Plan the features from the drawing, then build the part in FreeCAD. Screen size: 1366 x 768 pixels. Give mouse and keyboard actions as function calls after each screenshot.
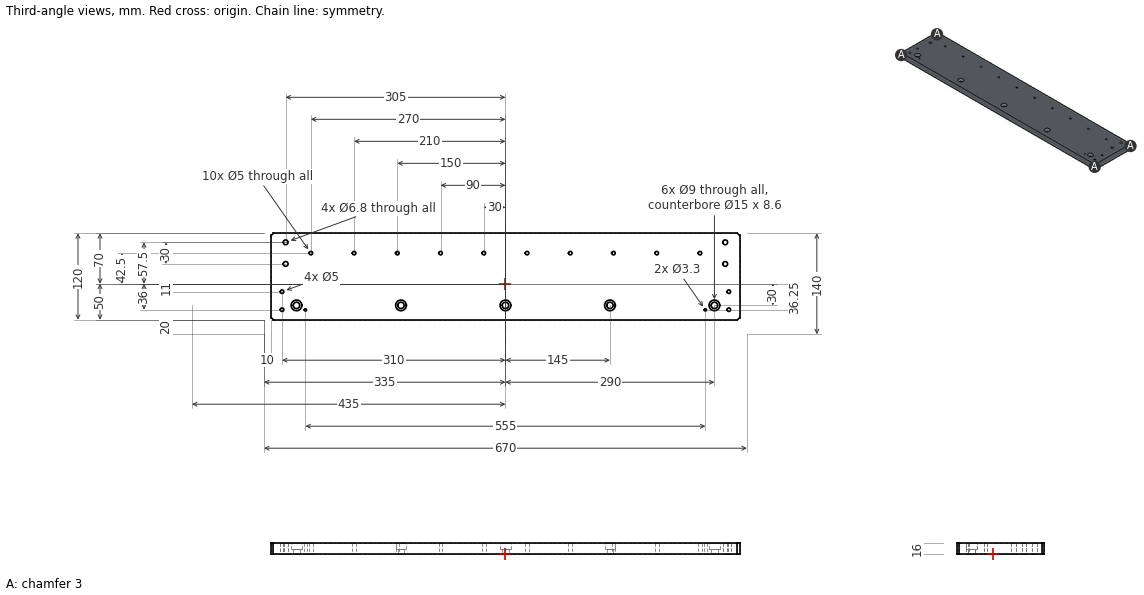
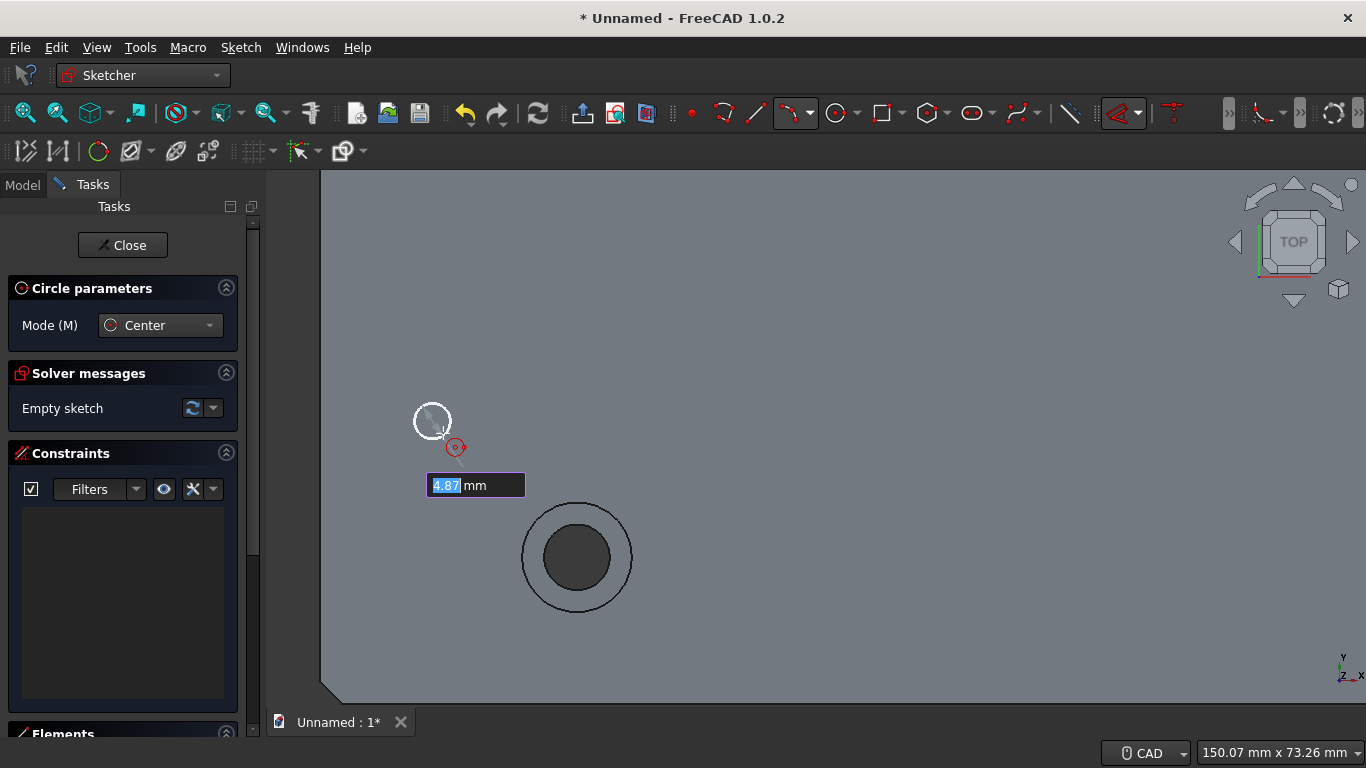
click(443, 431)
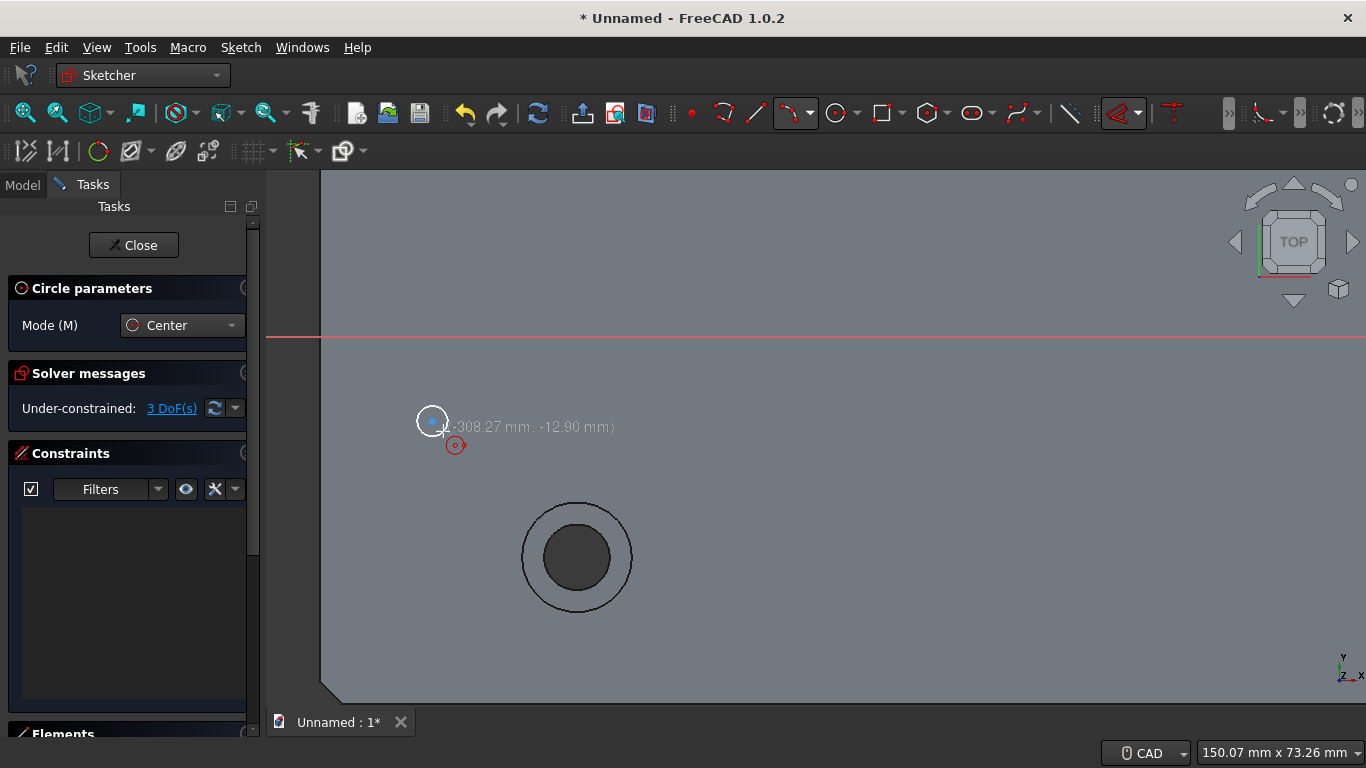
scroll(430, 601, up, 2)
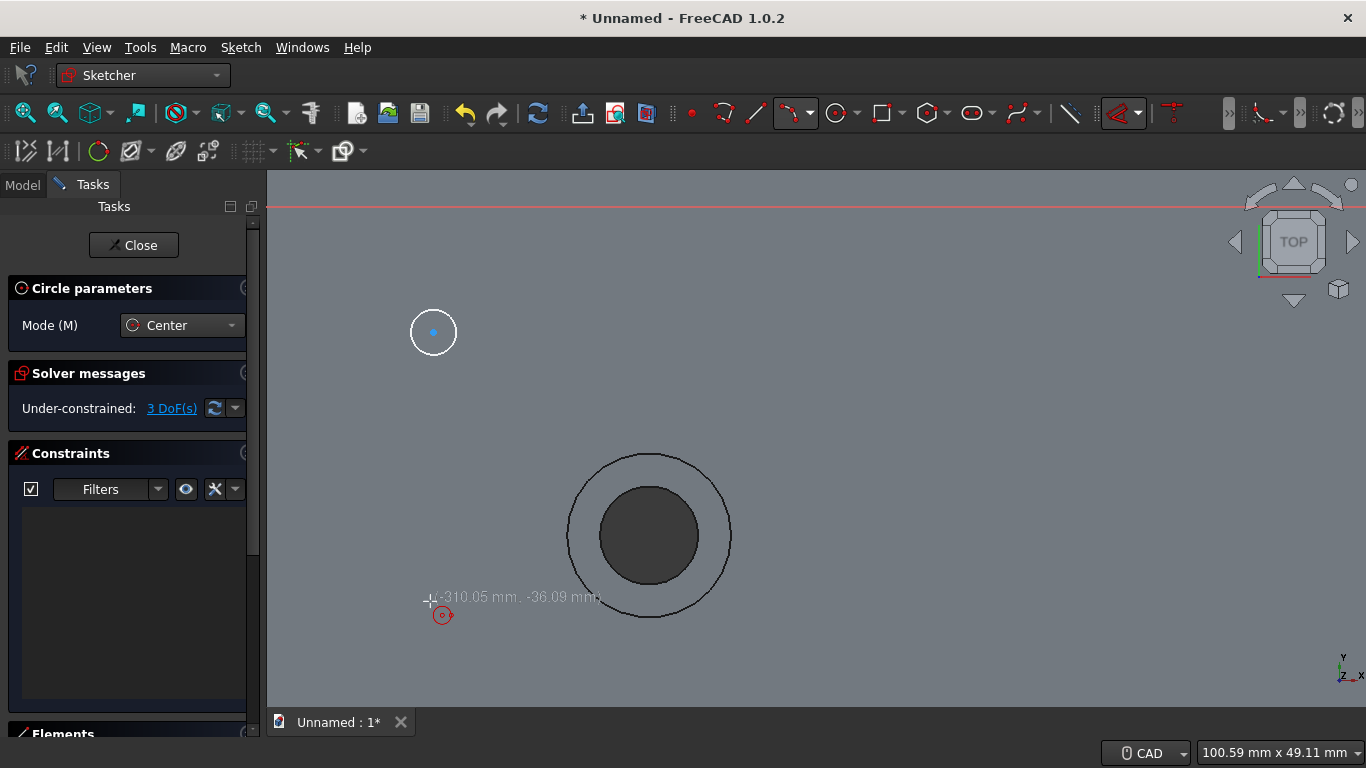
scroll(441, 441, down, 12)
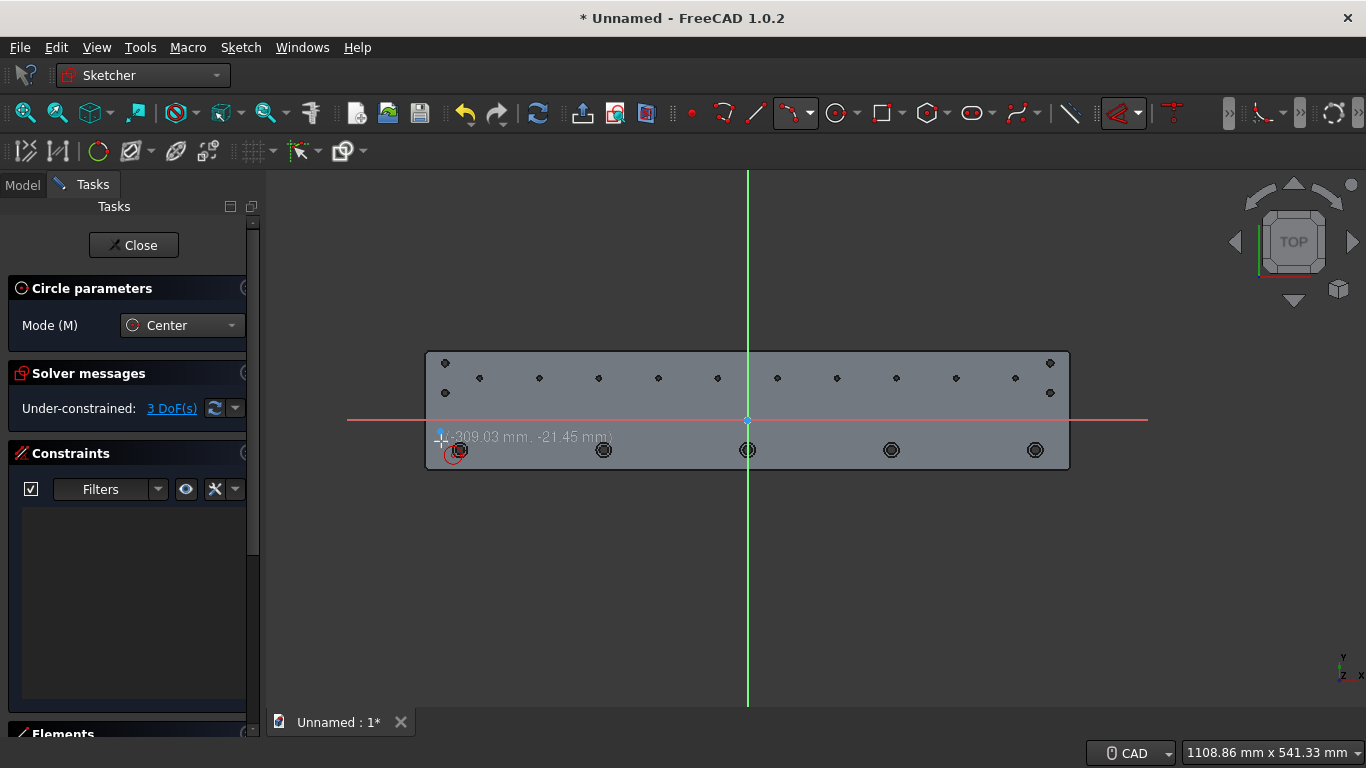
click(440, 456)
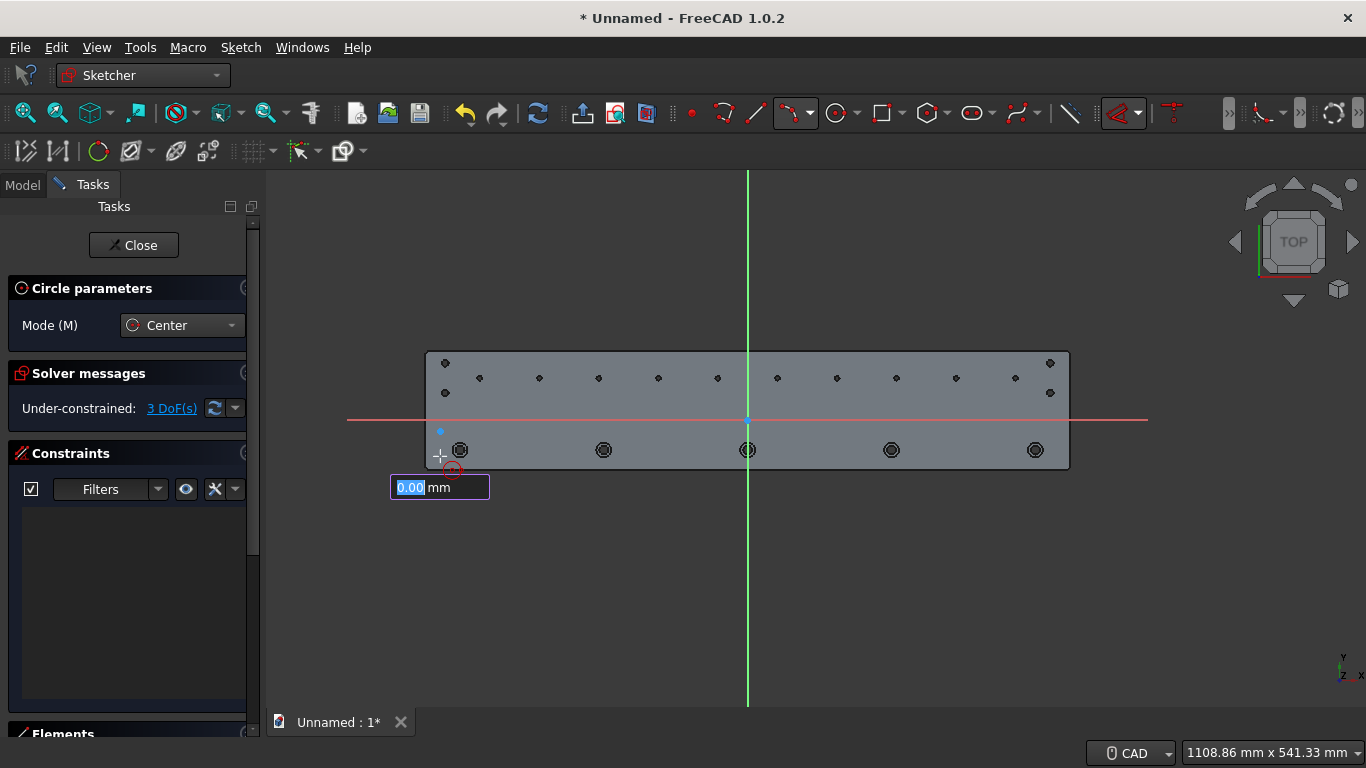
scroll(442, 454, up, 10)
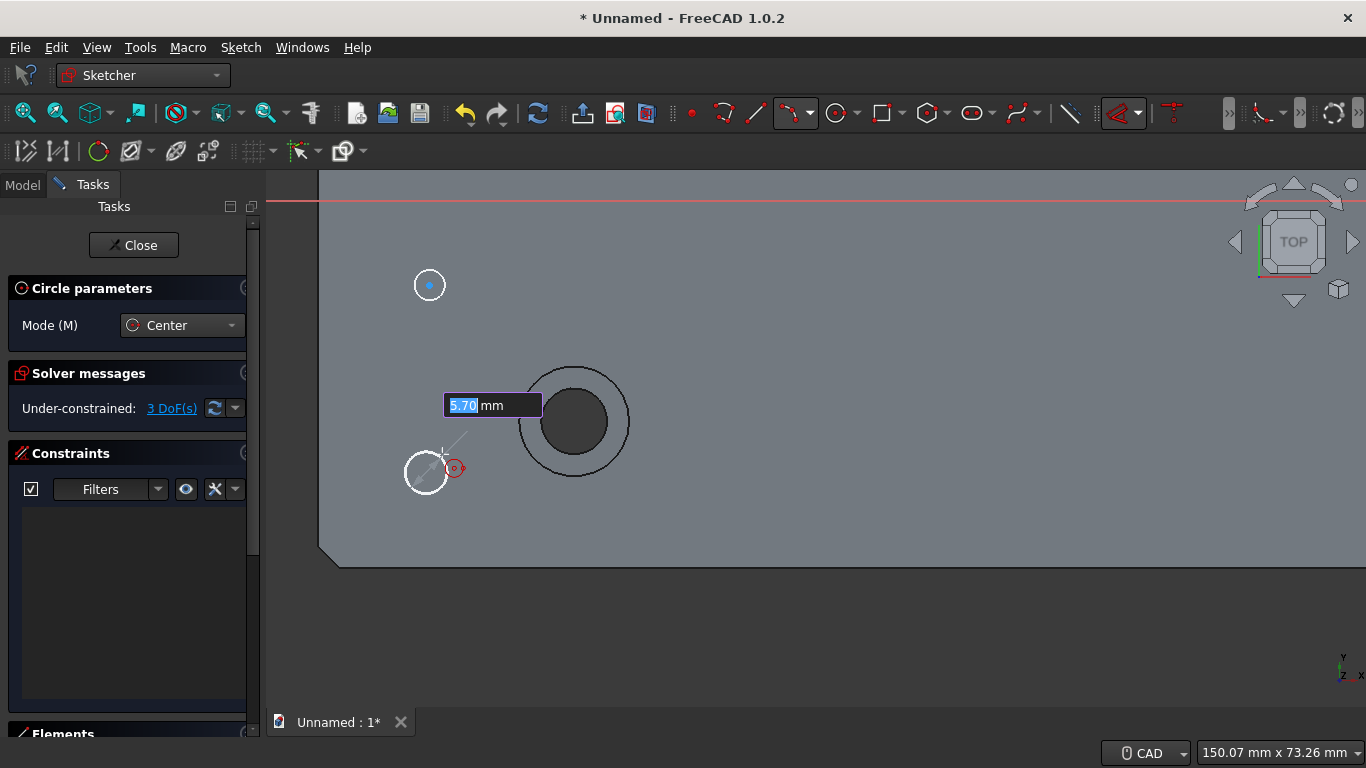
click(441, 452)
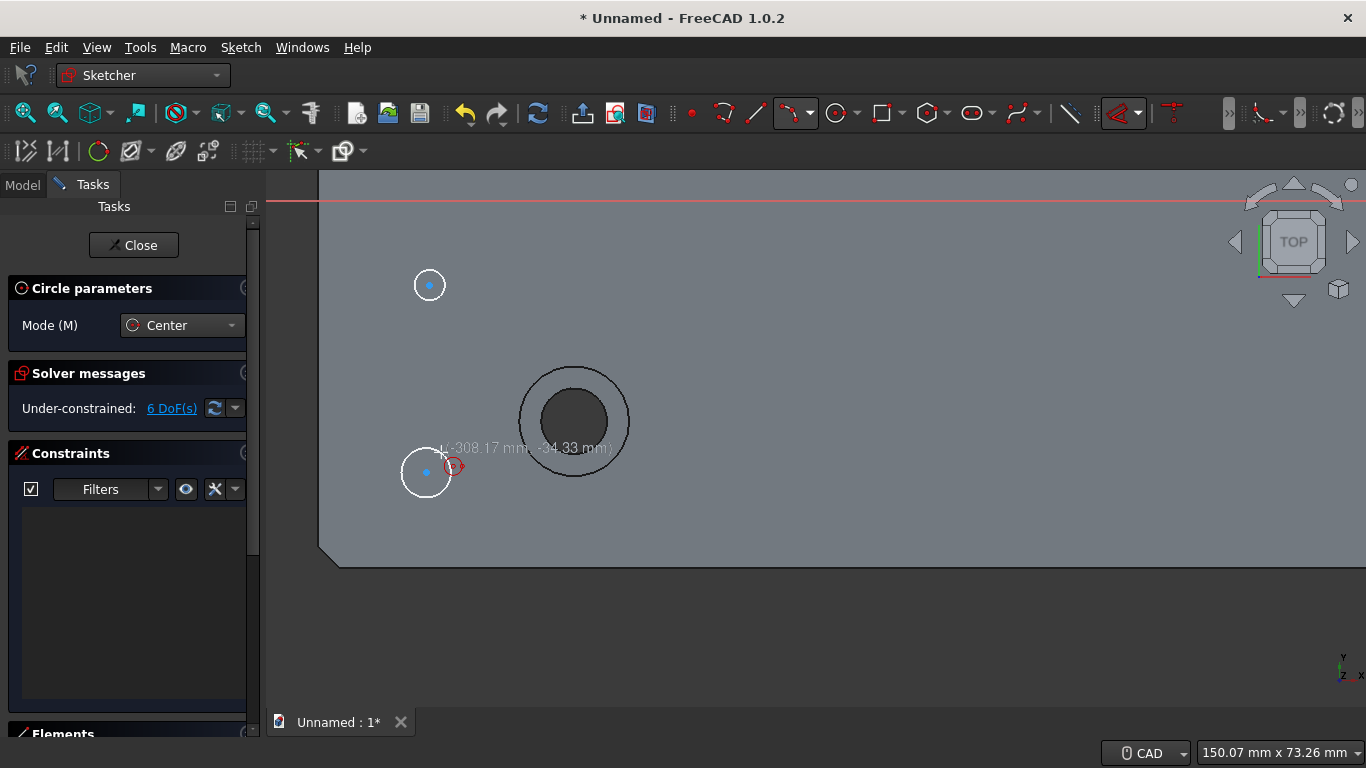
scroll(442, 454, down, 10)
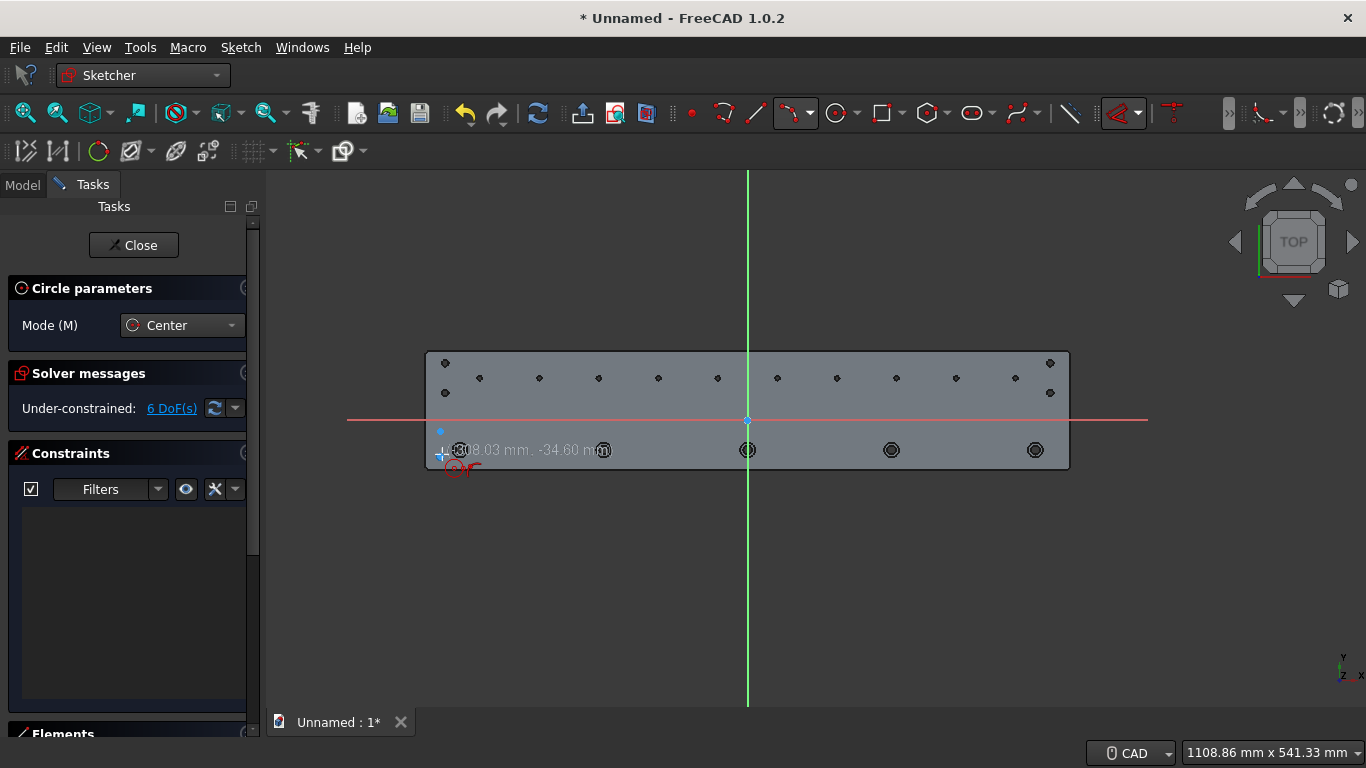
scroll(1055, 431, up, 12)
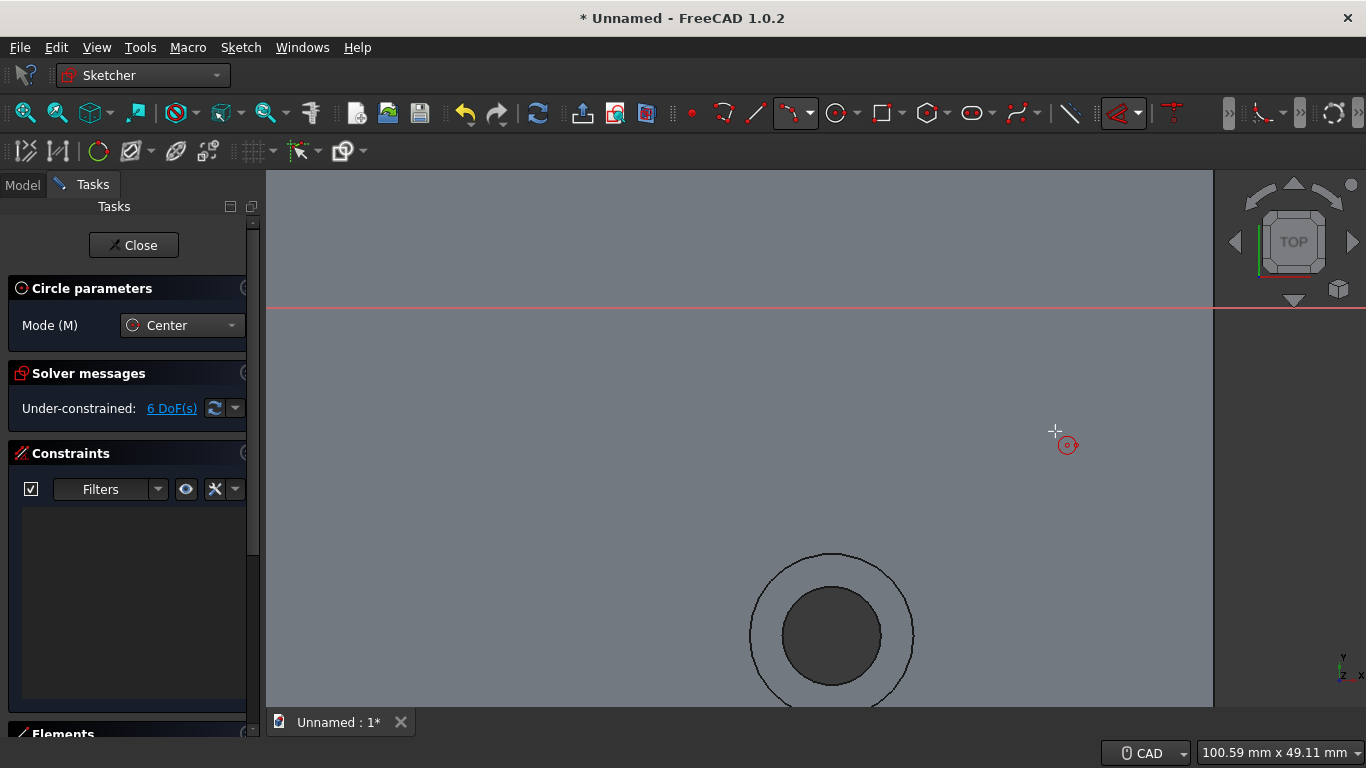
scroll(1055, 431, down, 12)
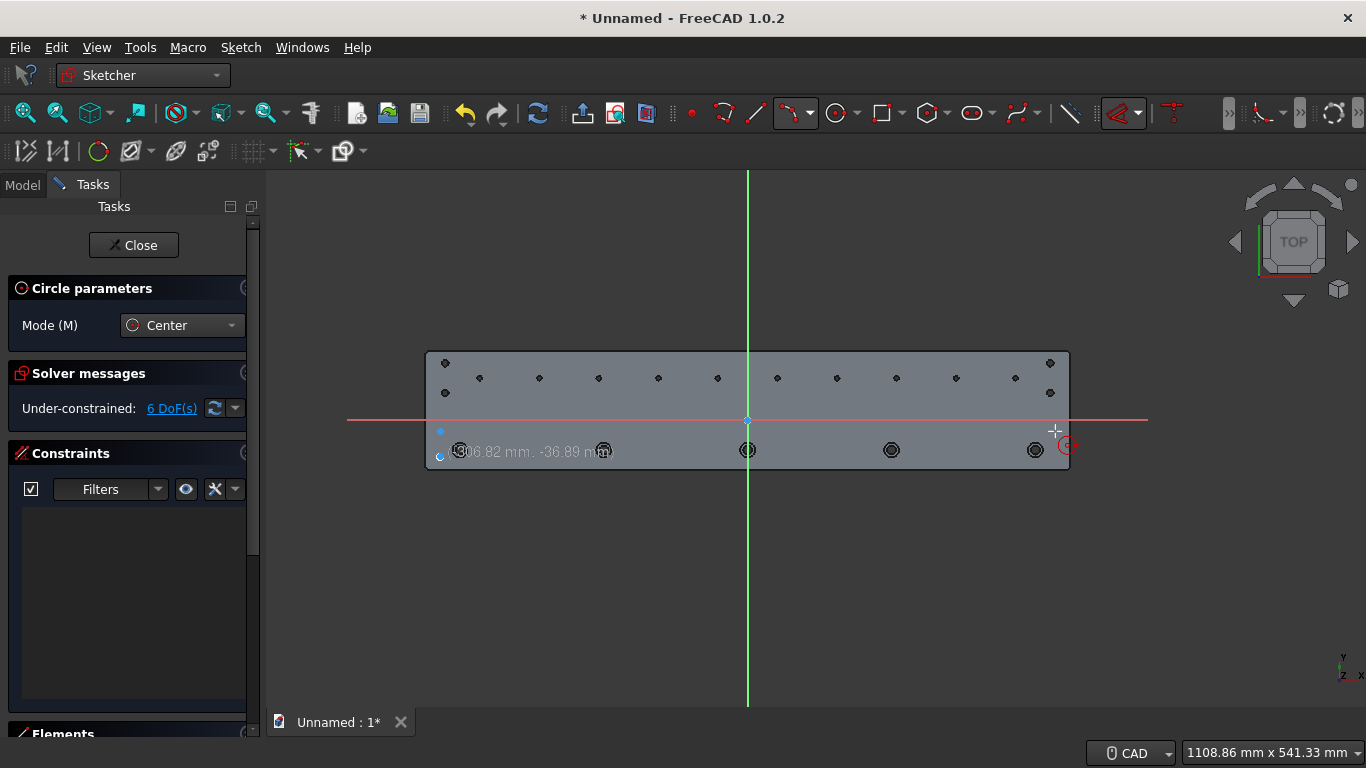
scroll(1055, 431, up, 2)